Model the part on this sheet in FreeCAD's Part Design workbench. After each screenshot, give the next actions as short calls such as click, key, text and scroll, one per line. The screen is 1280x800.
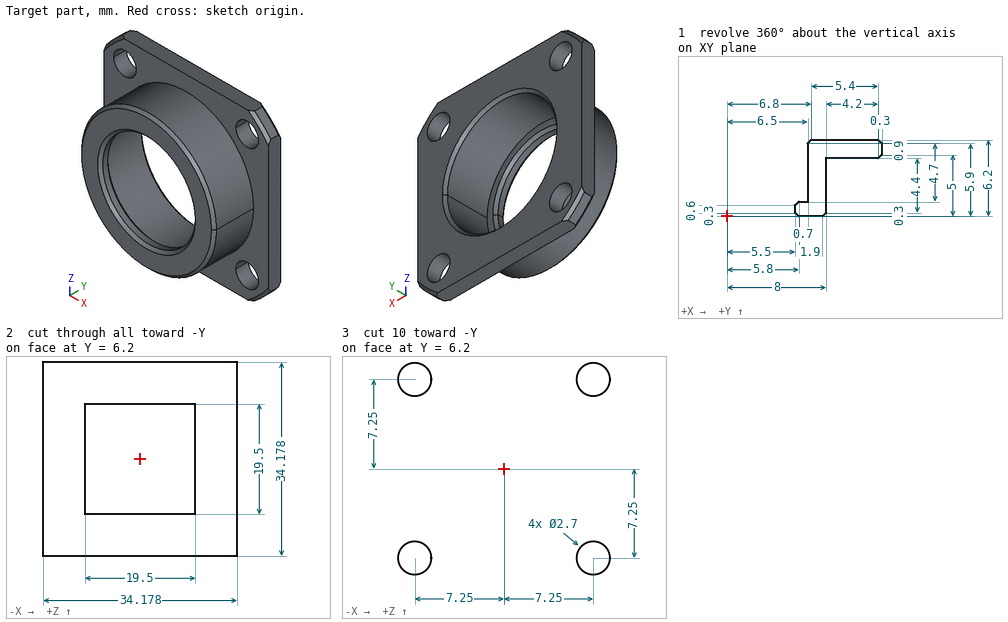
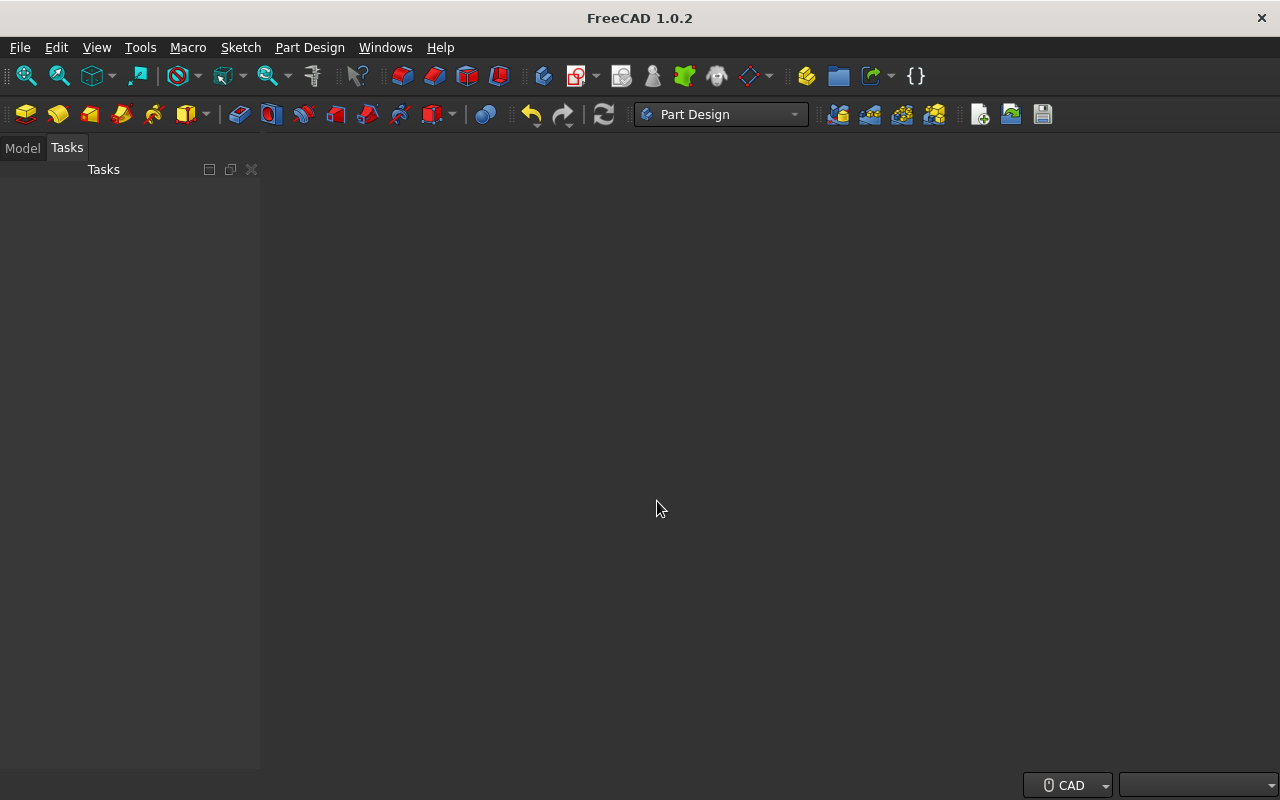
click(980, 112)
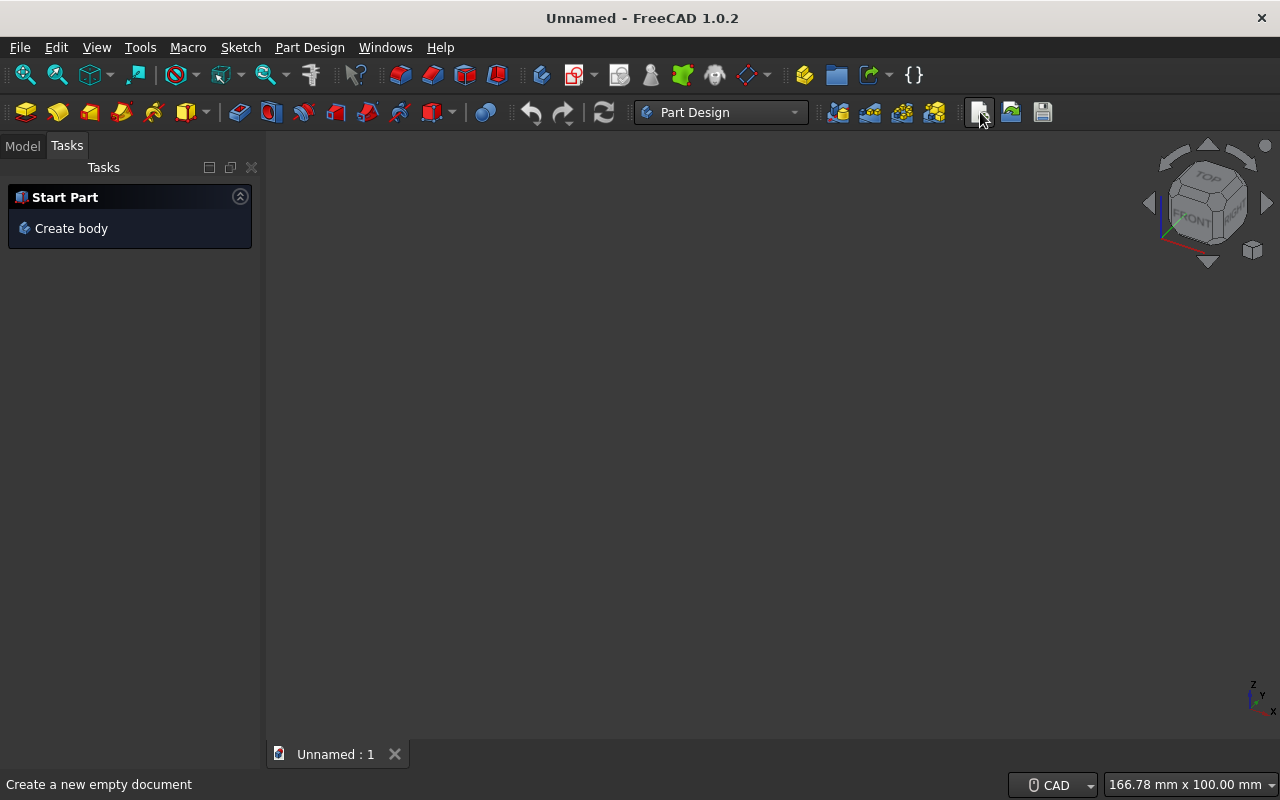
click(574, 76)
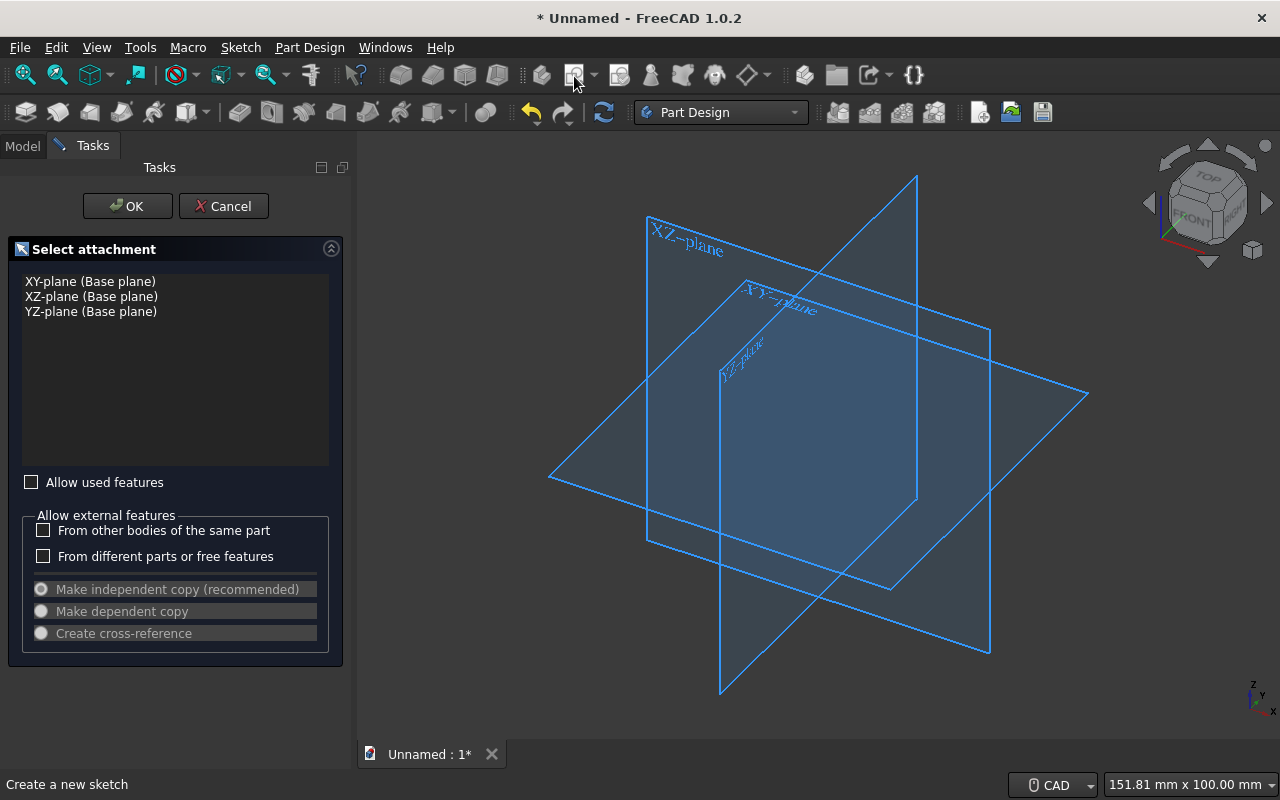
click(82, 282)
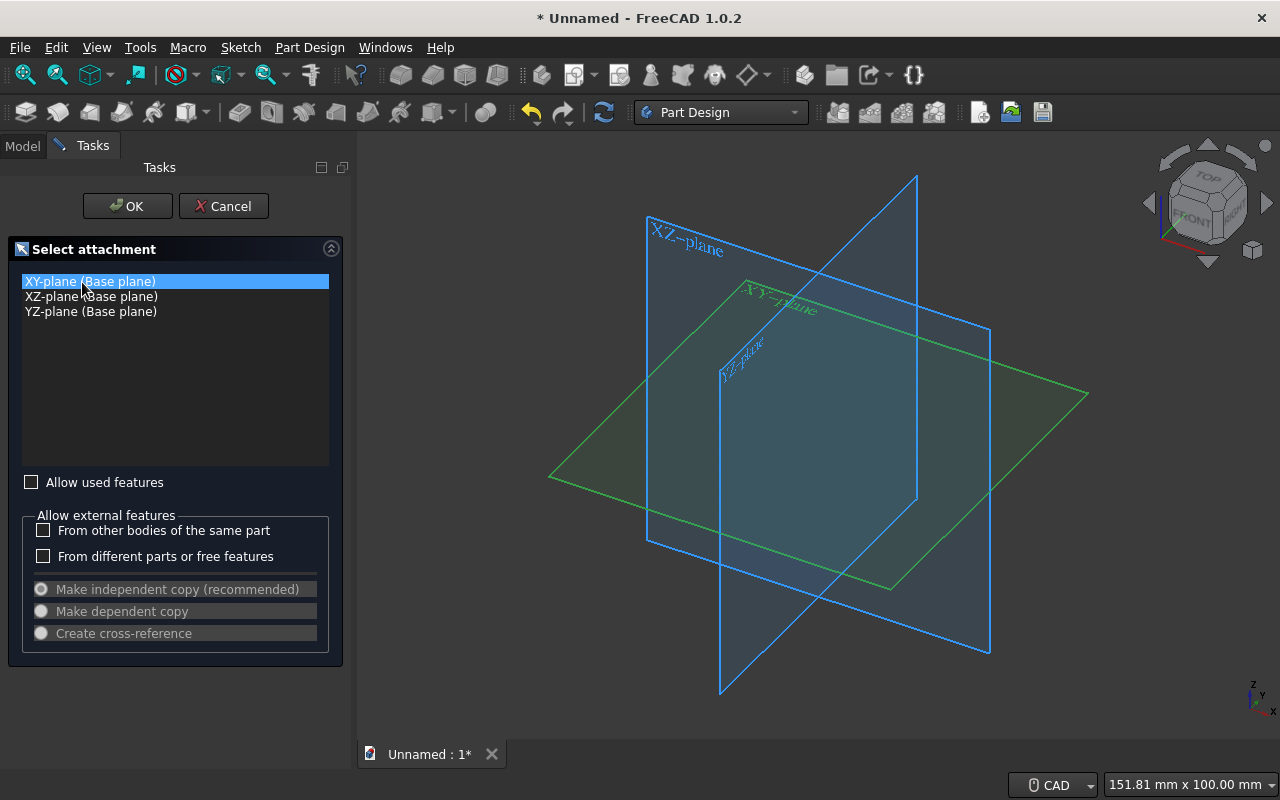
click(128, 206)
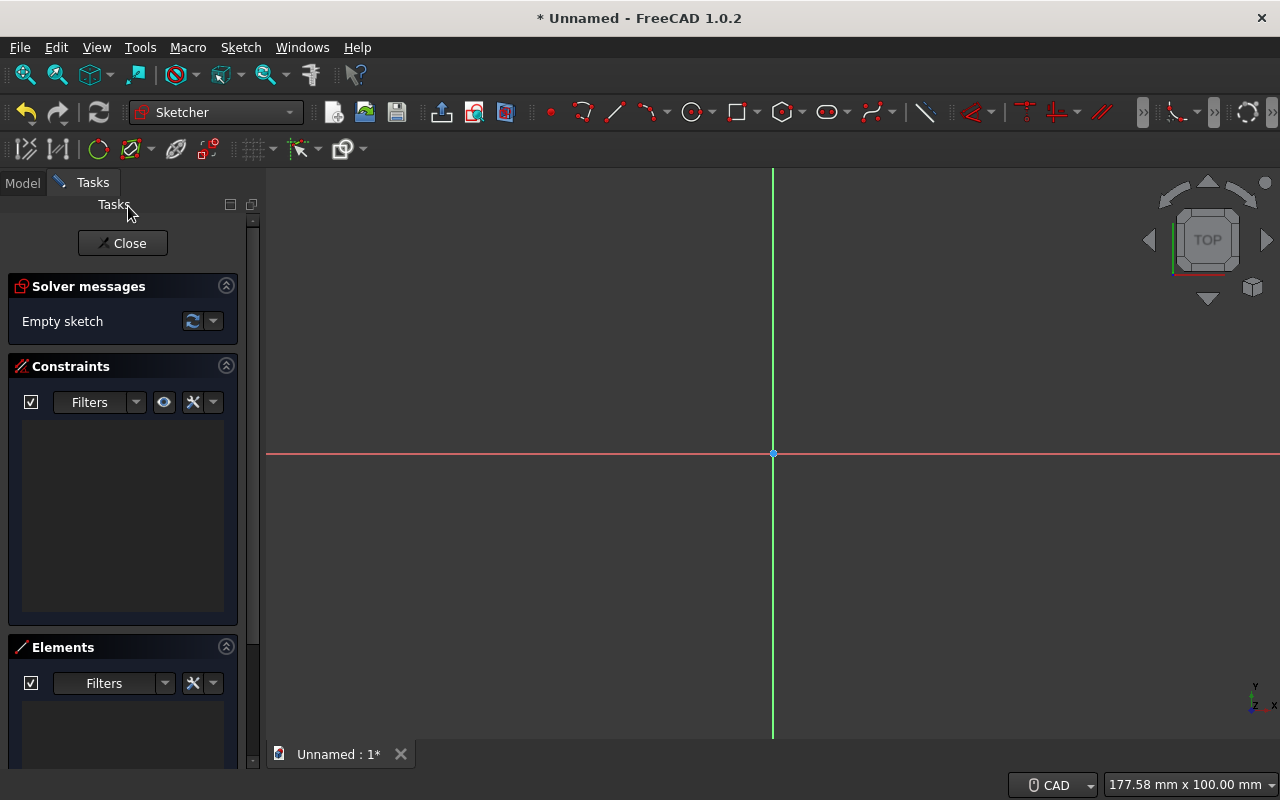
scroll(825, 433, up, 10)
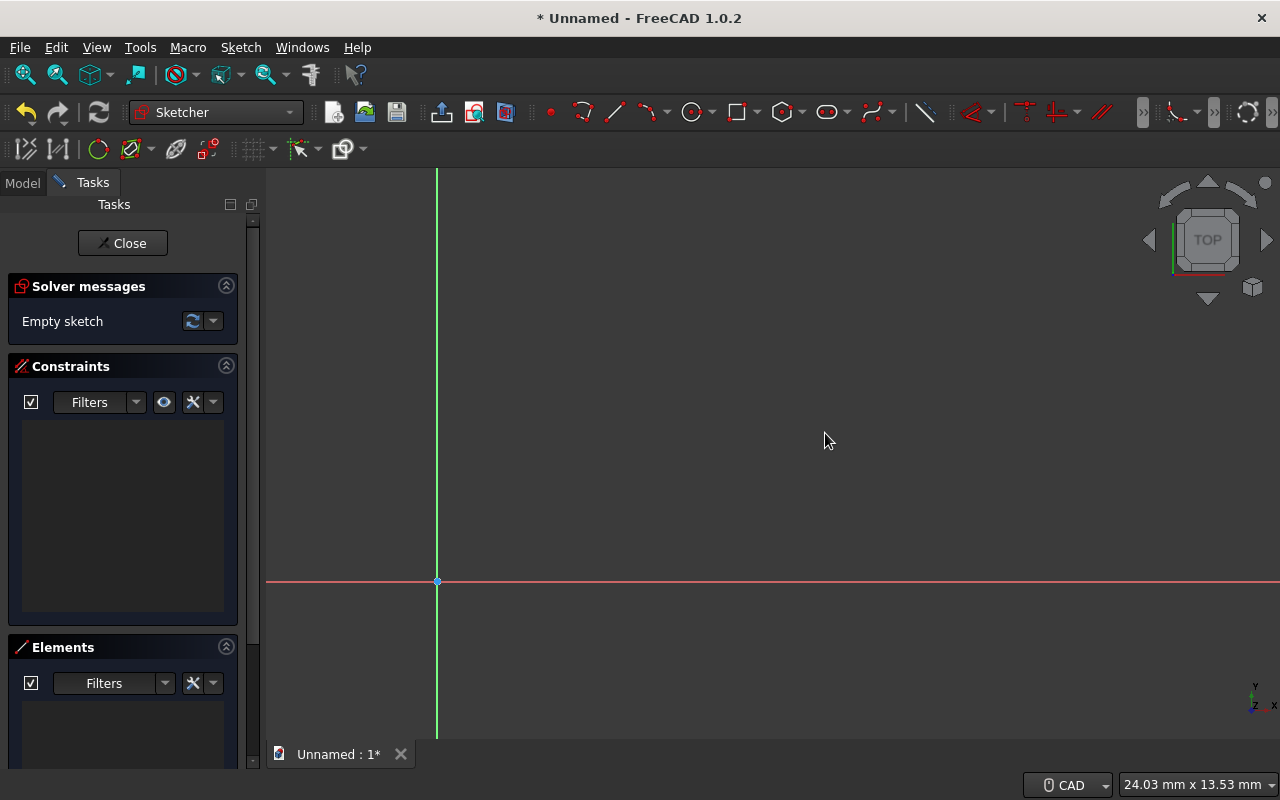
click(584, 112)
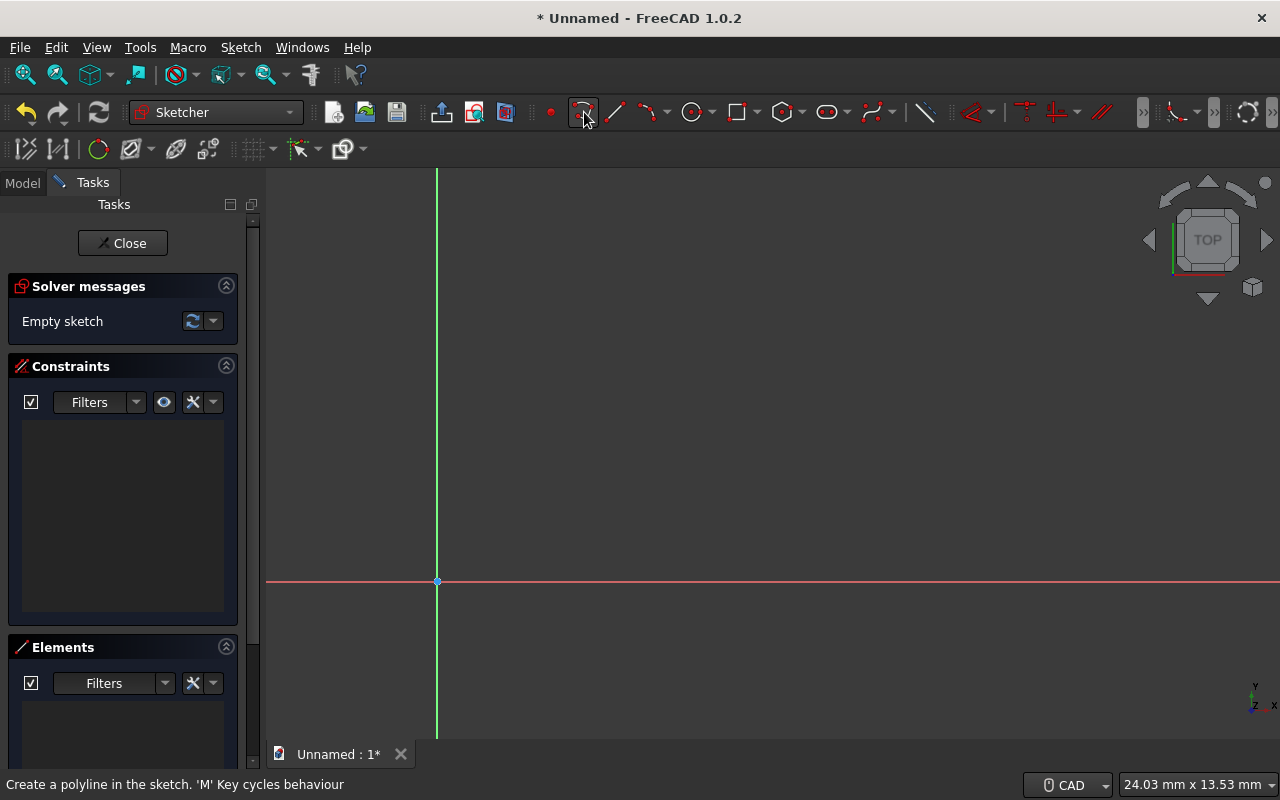
scroll(669, 569, up, 2)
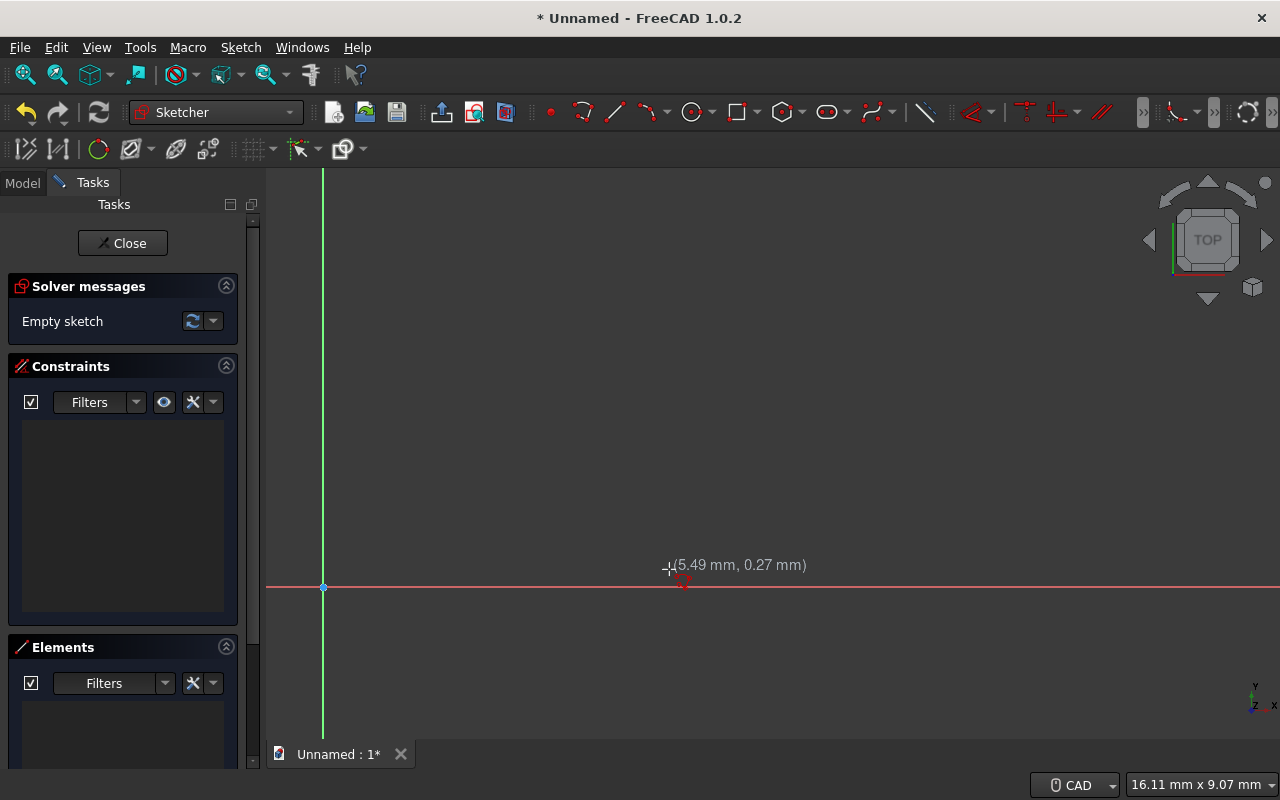
click(669, 568)
click(688, 587)
click(808, 578)
click(827, 568)
click(827, 291)
click(1091, 291)
click(1110, 273)
click(1110, 216)
click(1091, 197)
click(751, 197)
click(732, 216)
click(732, 512)
click(688, 512)
click(669, 531)
click(669, 569)
key(Escape)
key(Escape)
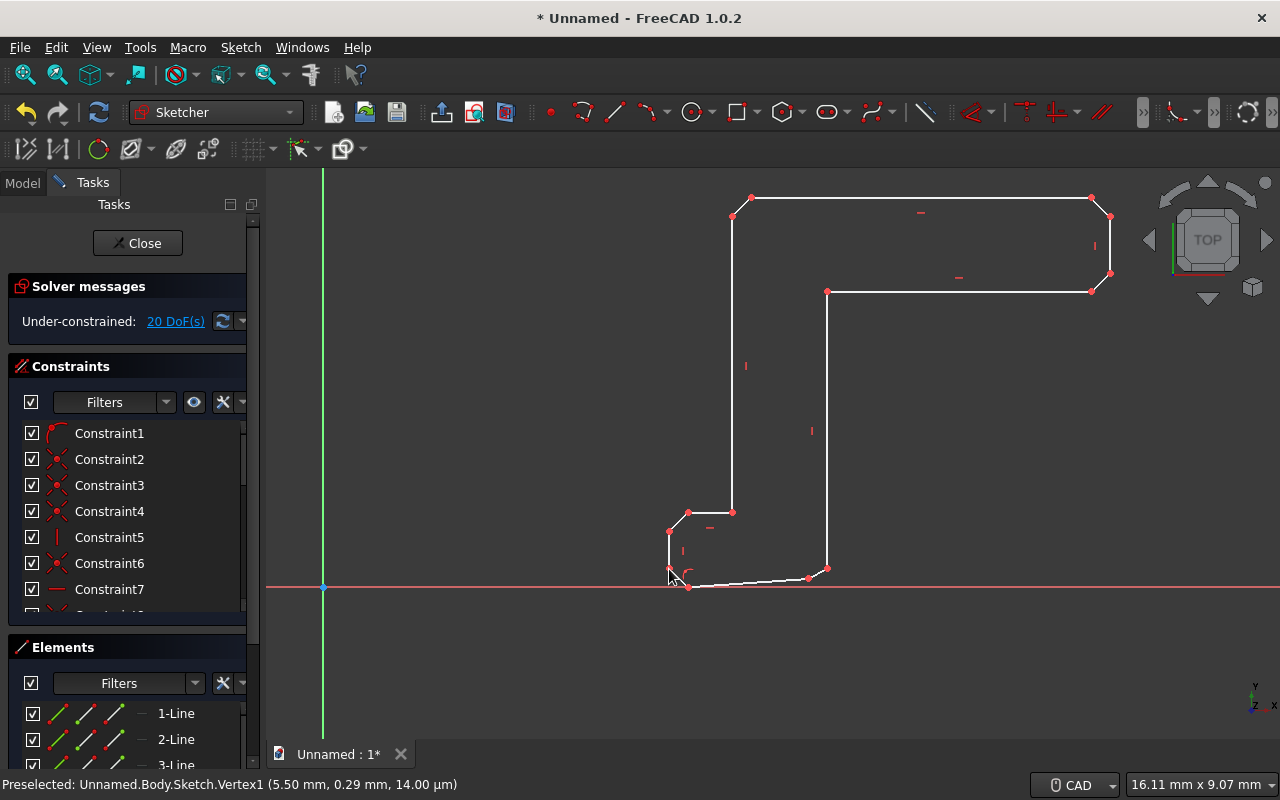
click(724, 585)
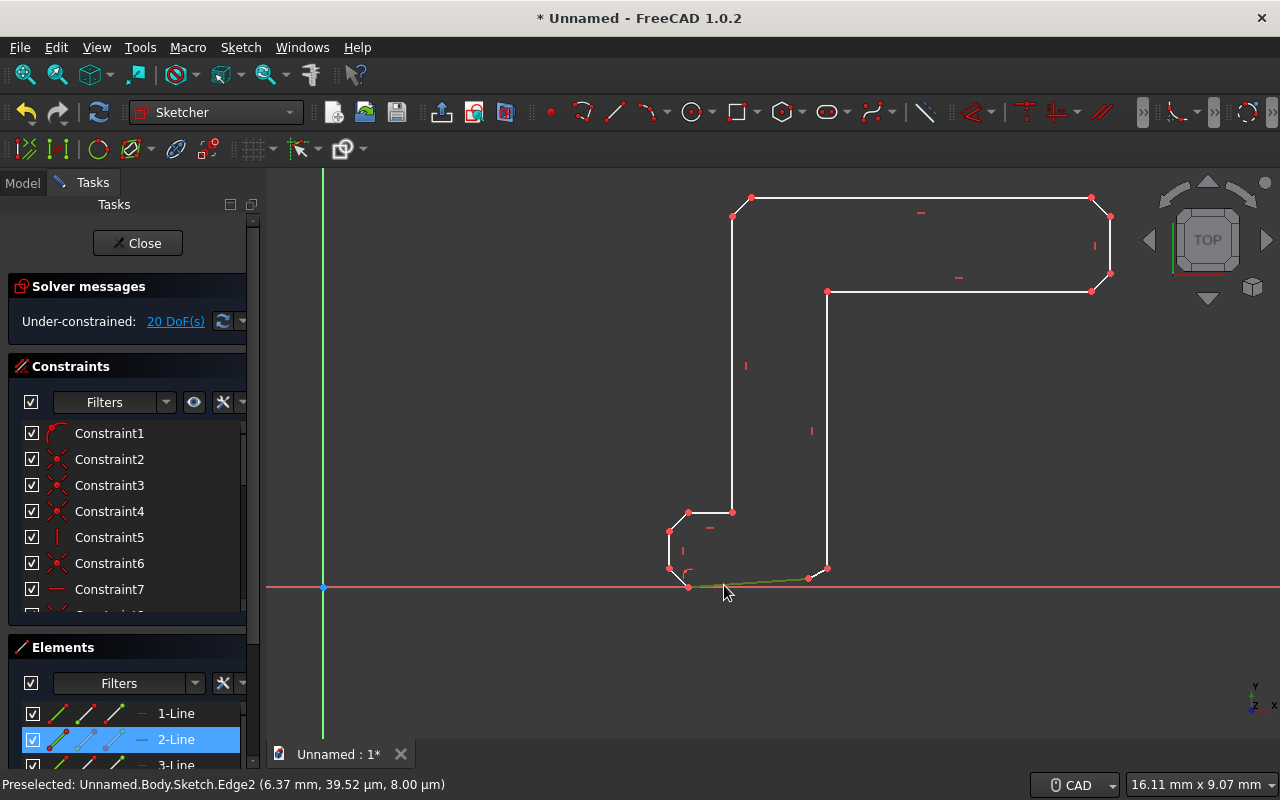
click(1080, 112)